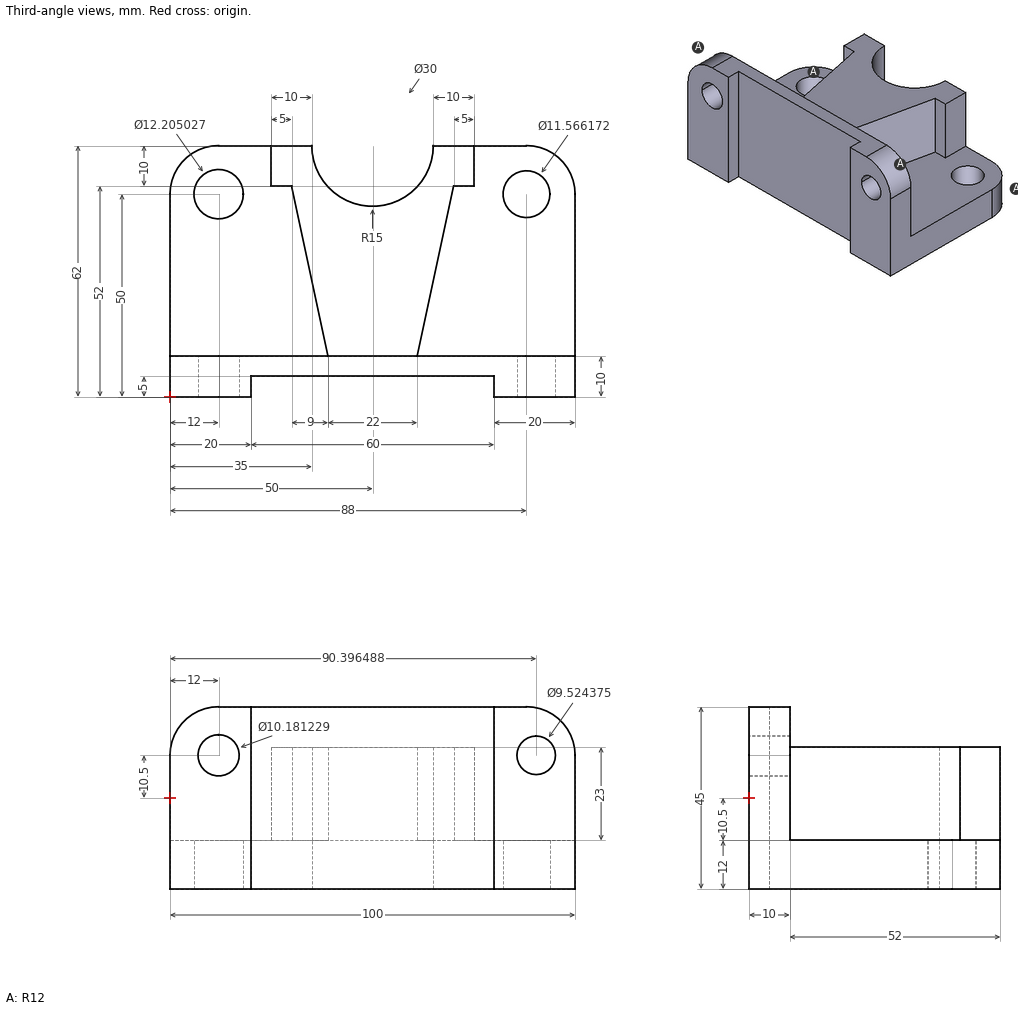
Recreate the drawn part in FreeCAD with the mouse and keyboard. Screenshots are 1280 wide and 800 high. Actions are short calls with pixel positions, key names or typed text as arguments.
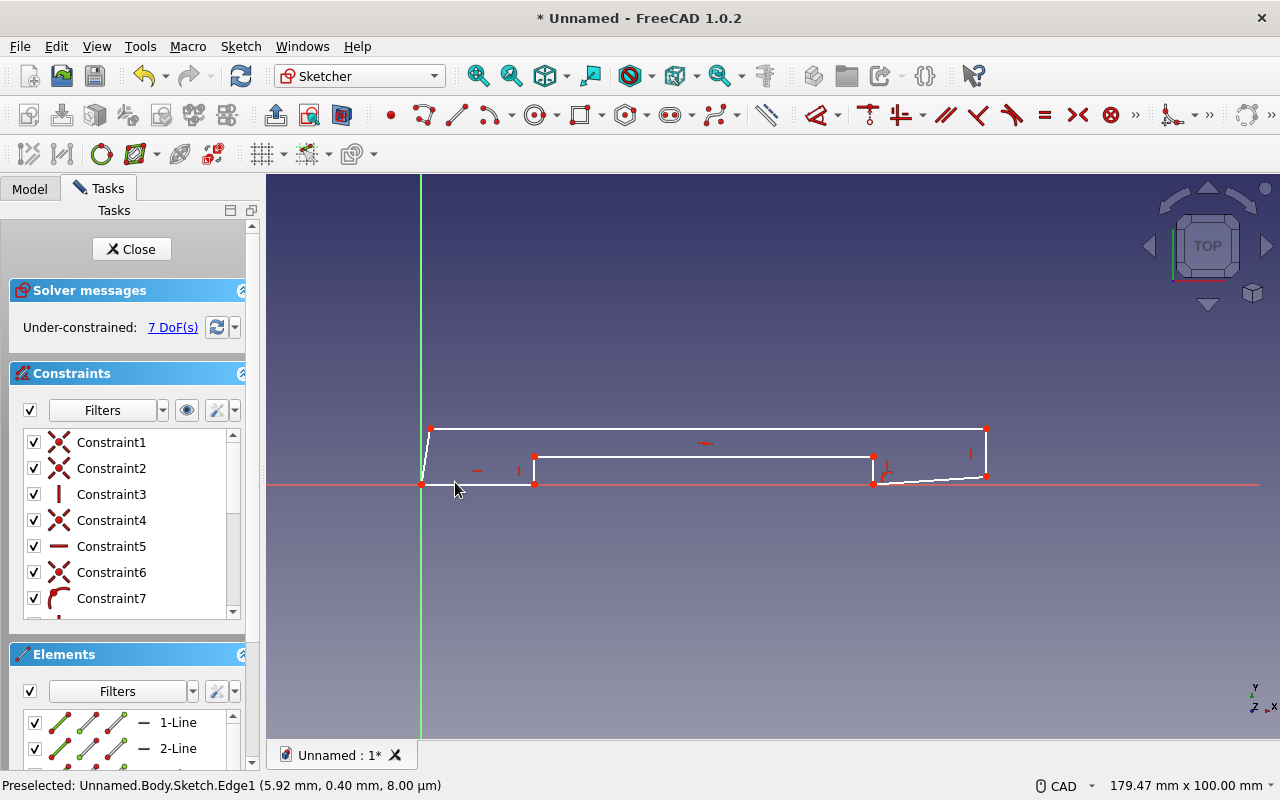
click(907, 482)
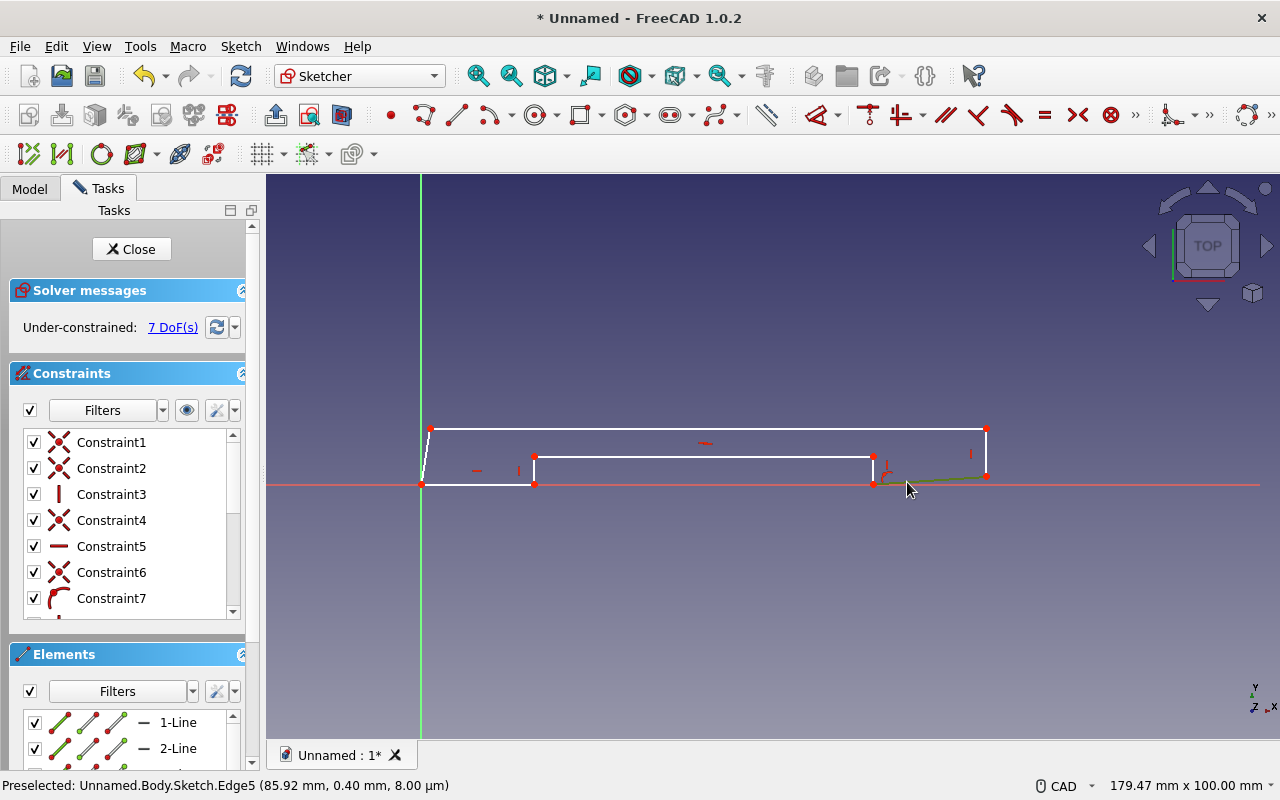
key(h)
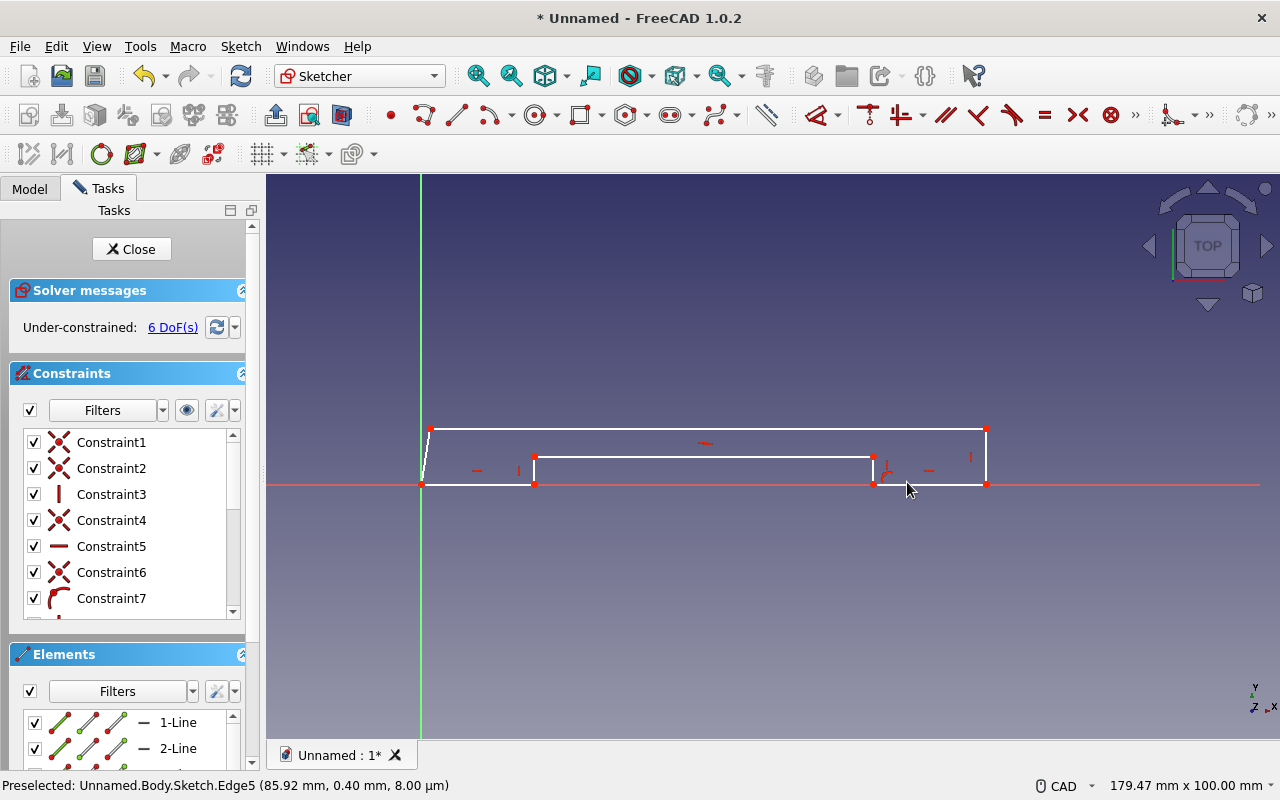
click(424, 468)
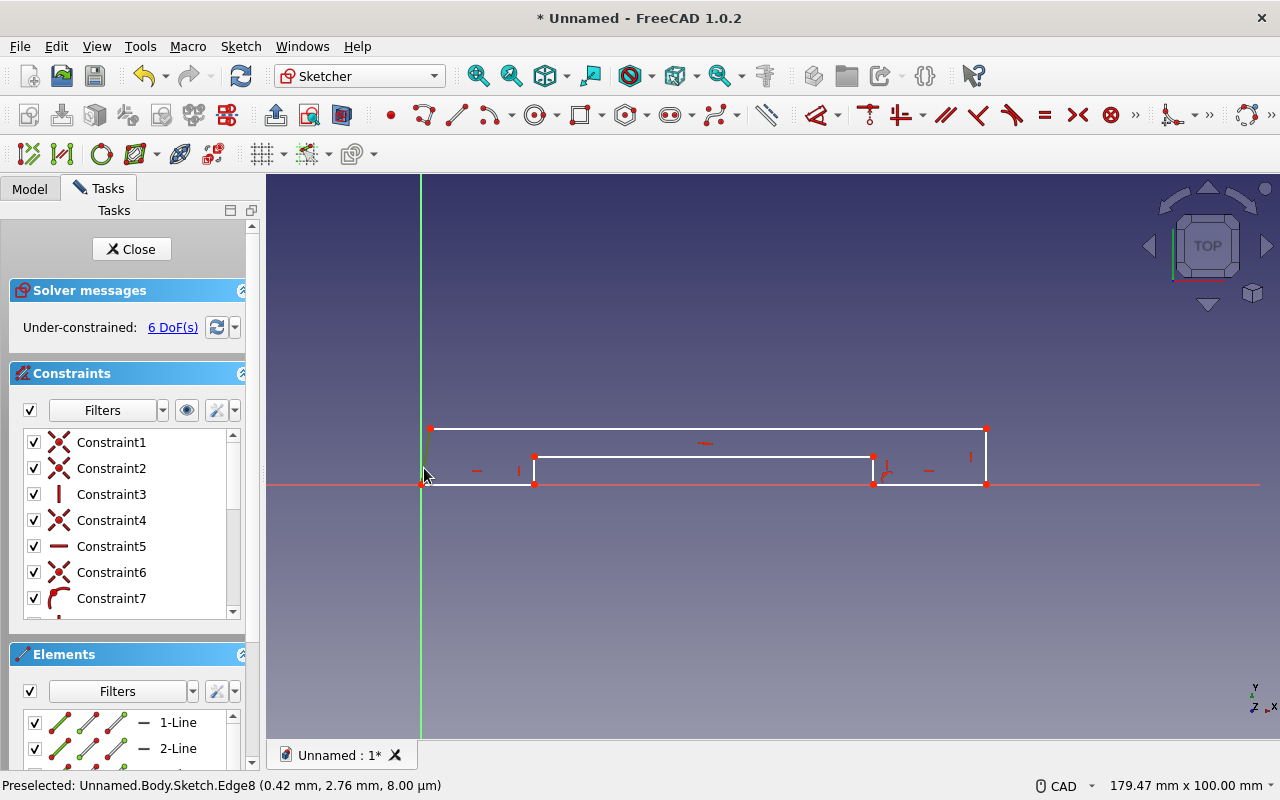
click(922, 116)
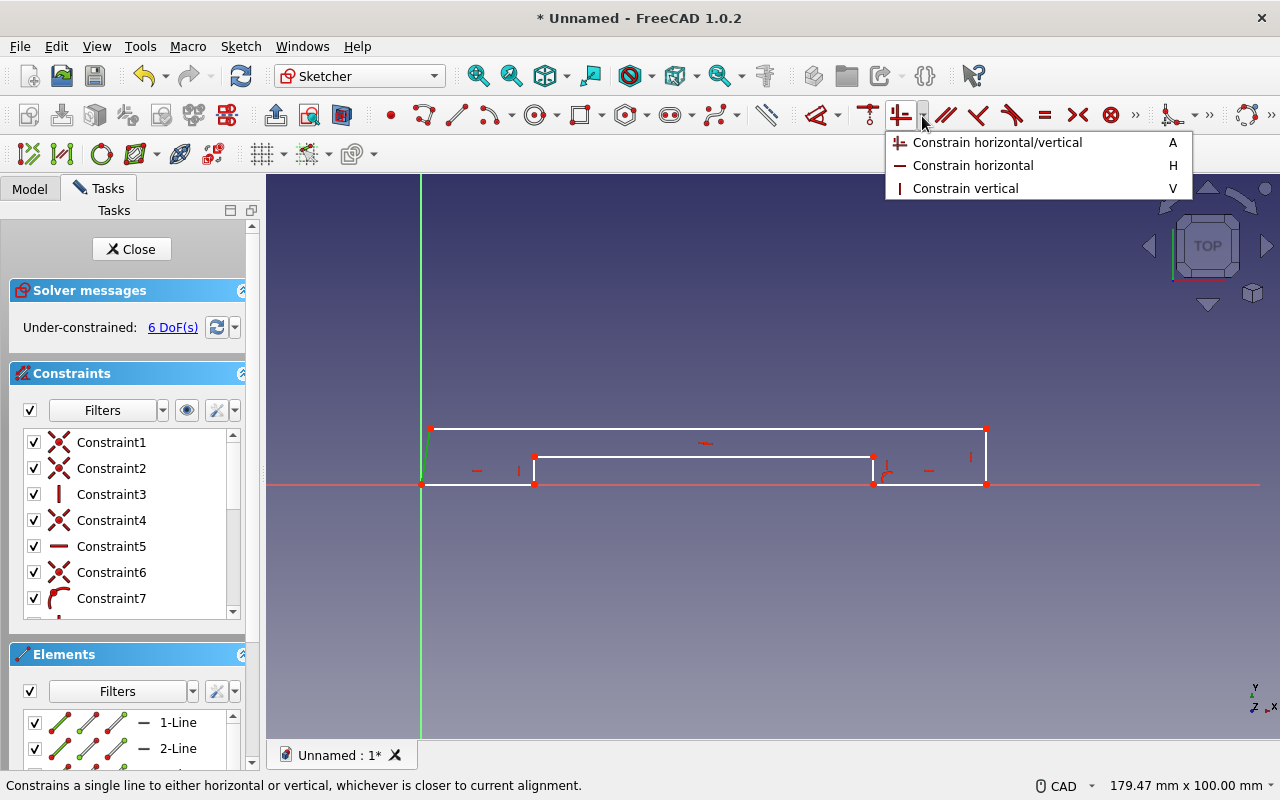
click(1039, 188)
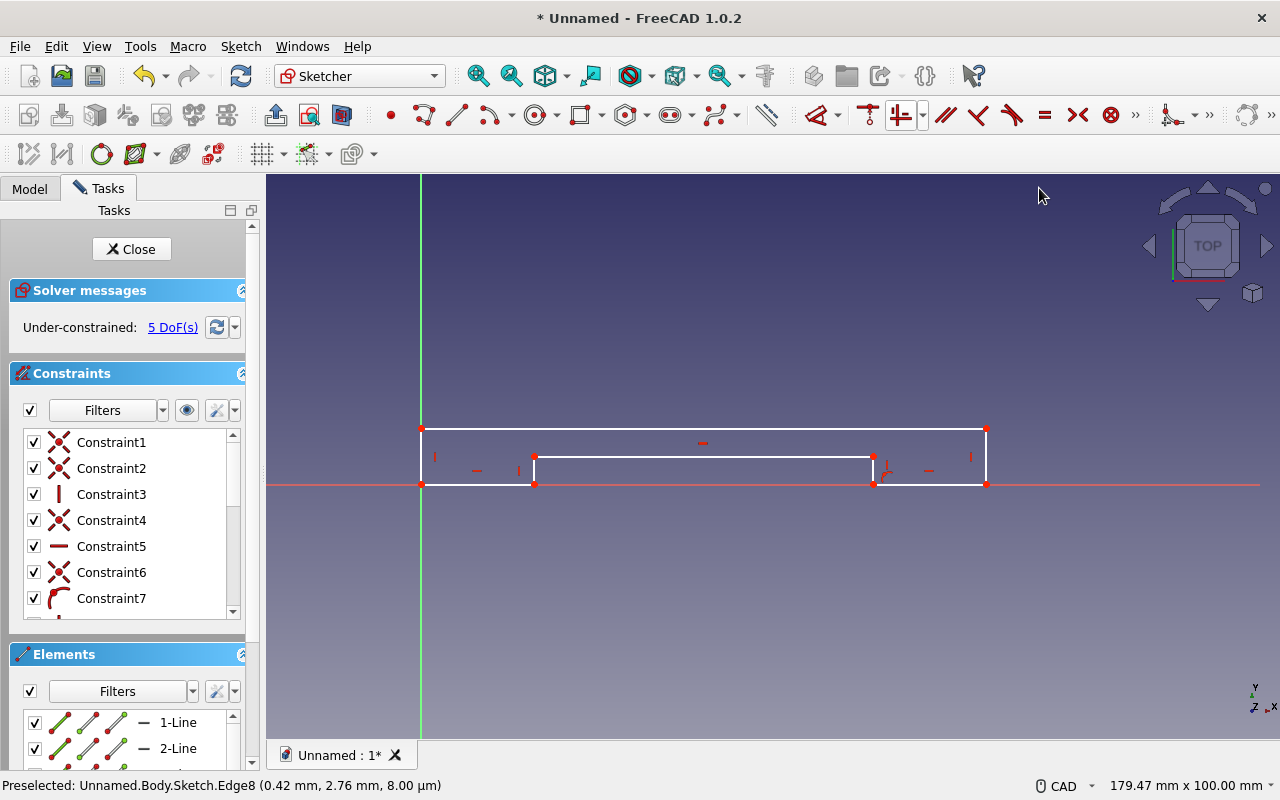
scroll(534, 474, up, 2)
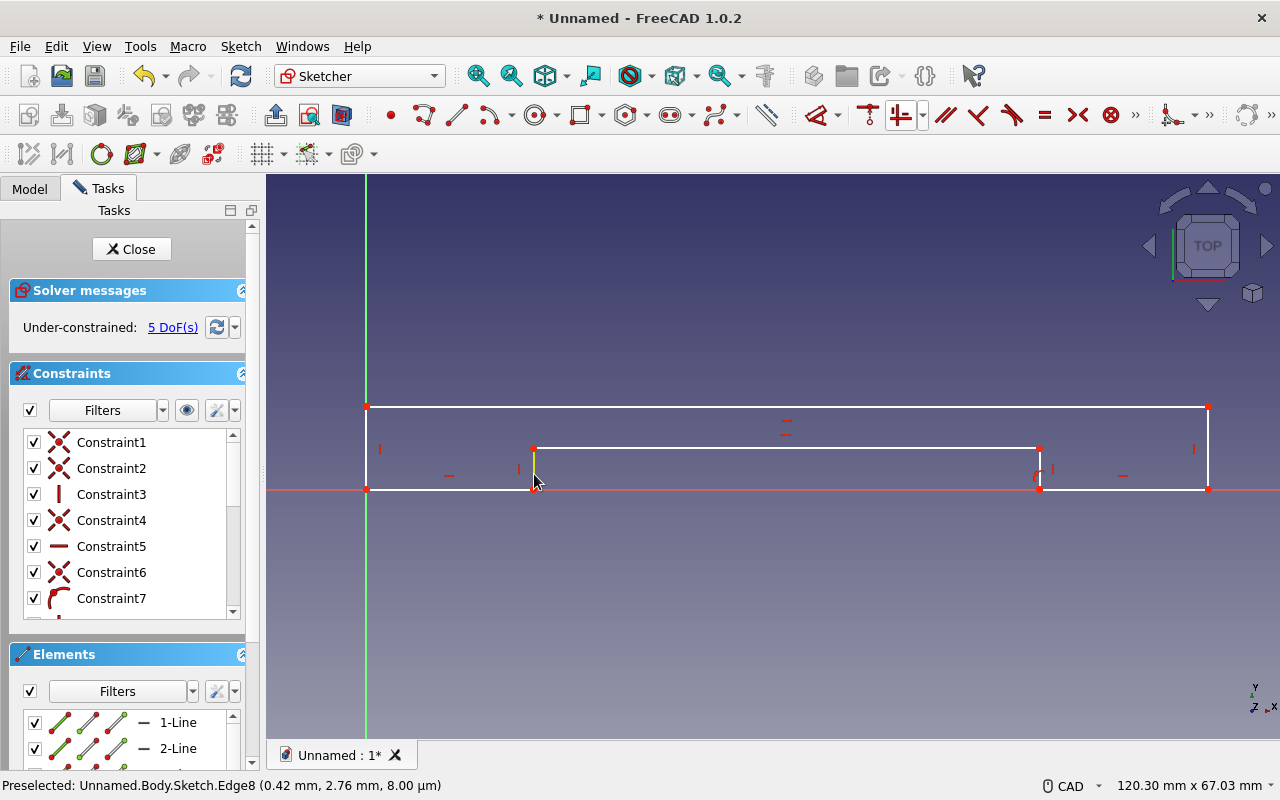
click(534, 473)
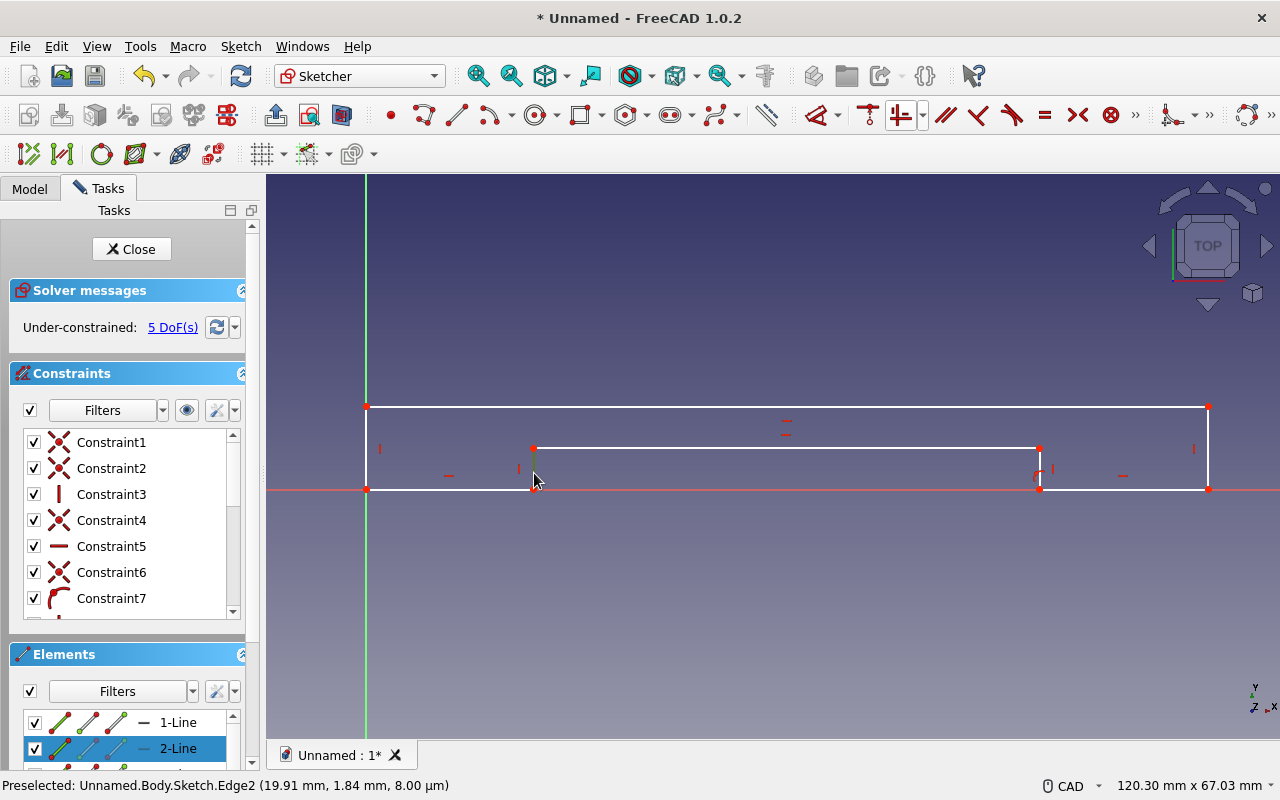
key(i)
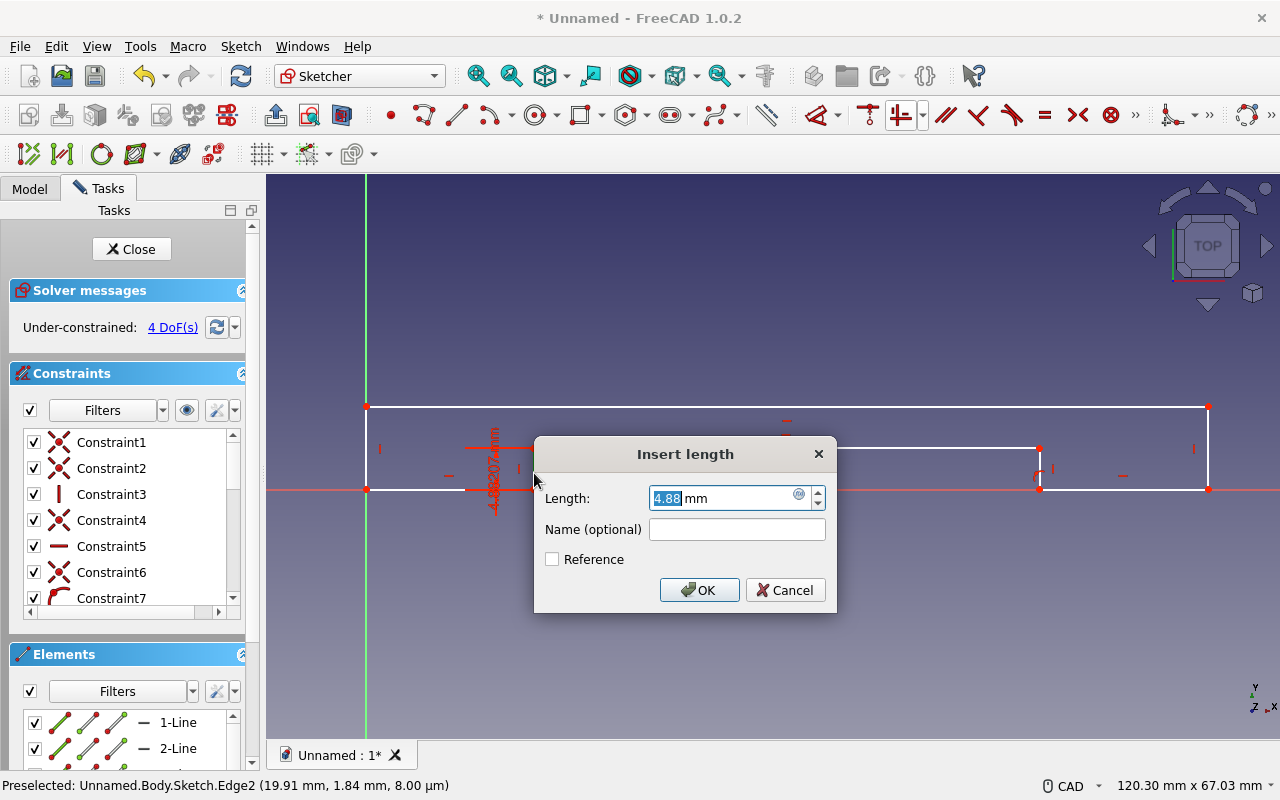
text(5)
key(Return)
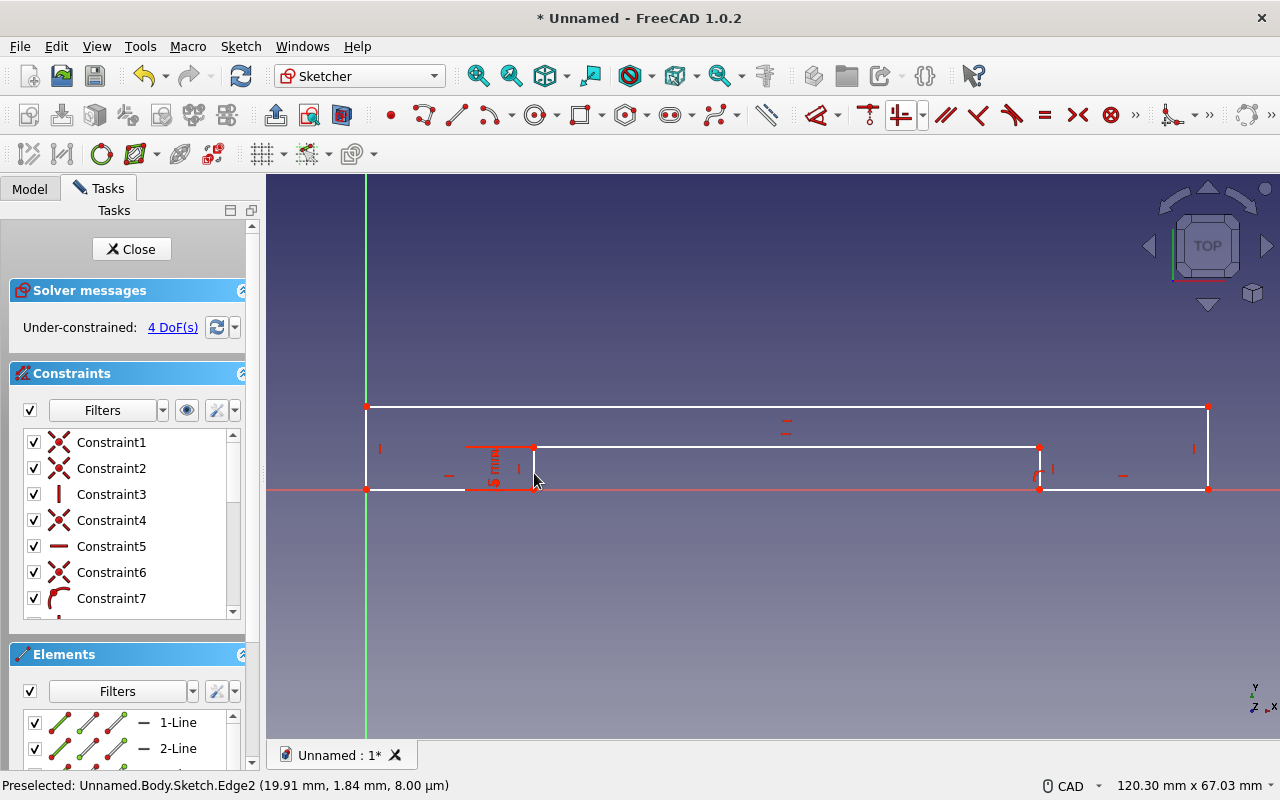
click(416, 490)